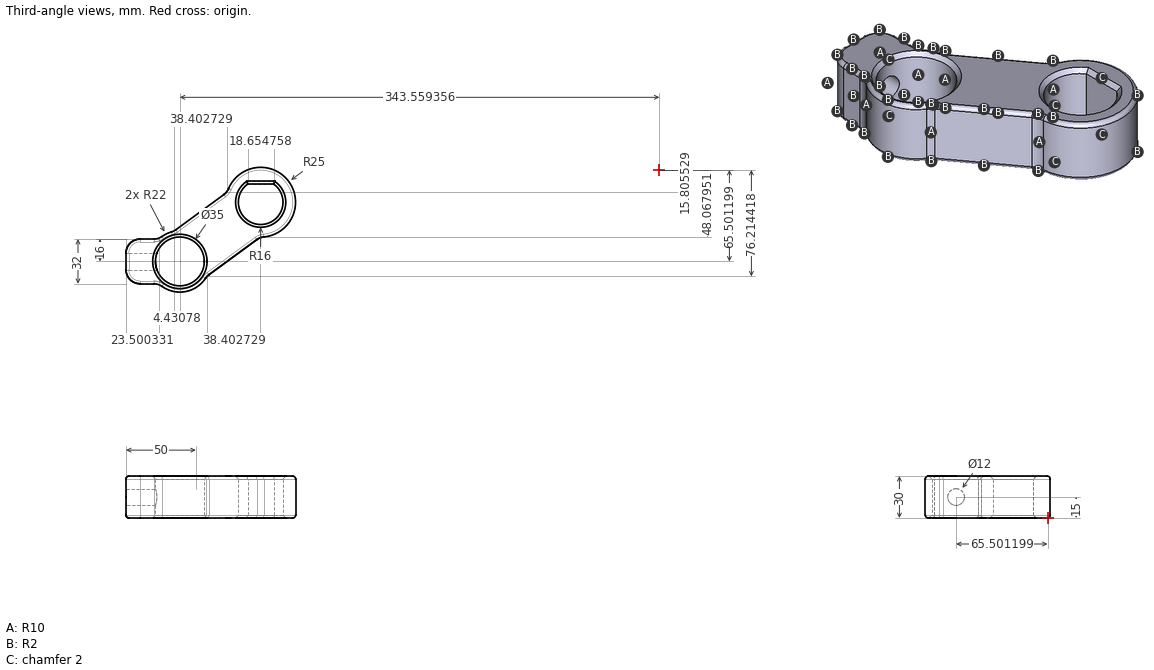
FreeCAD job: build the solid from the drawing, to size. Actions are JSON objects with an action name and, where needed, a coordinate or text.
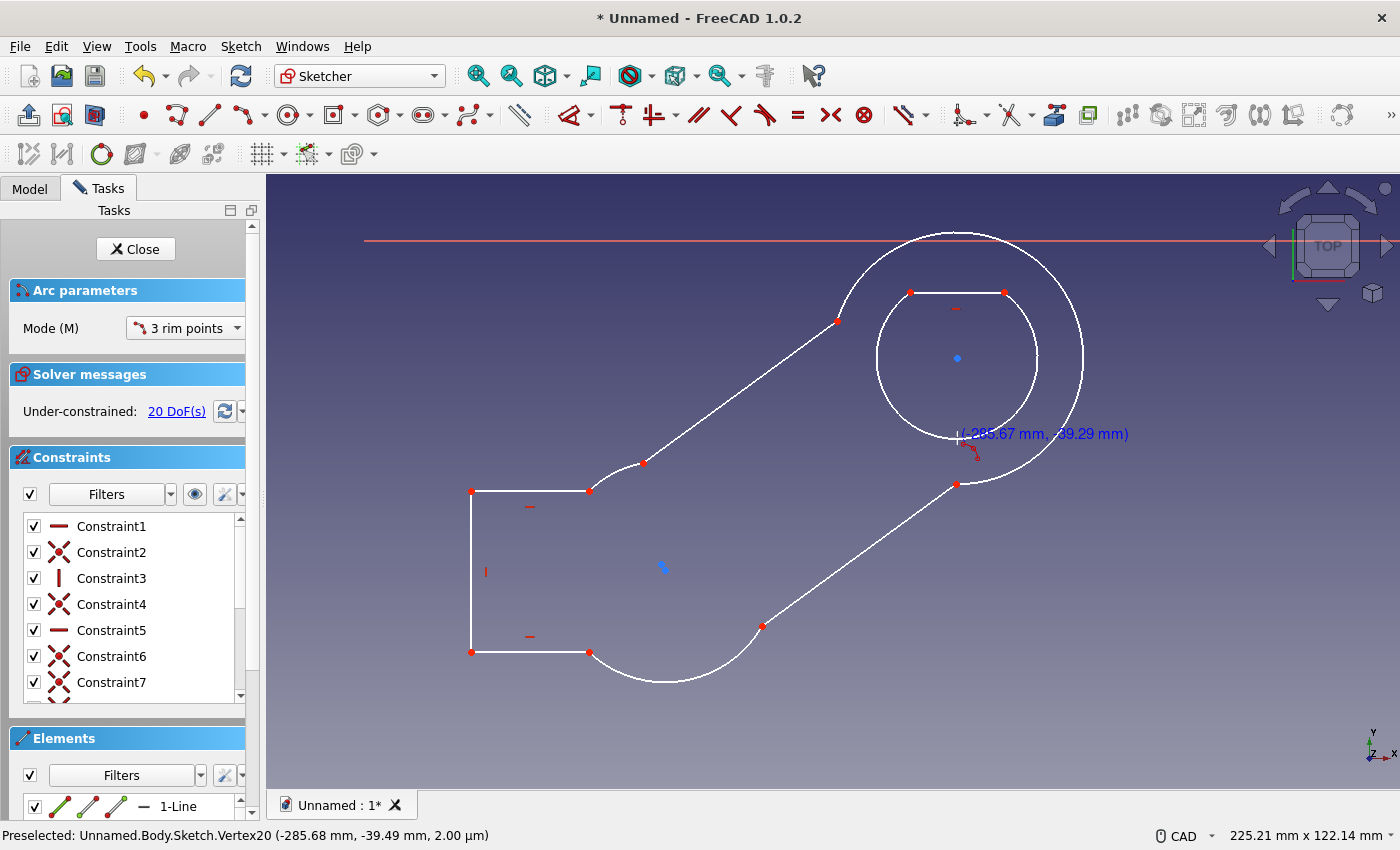
{"action": "left_click", "coordinate": [288, 116]}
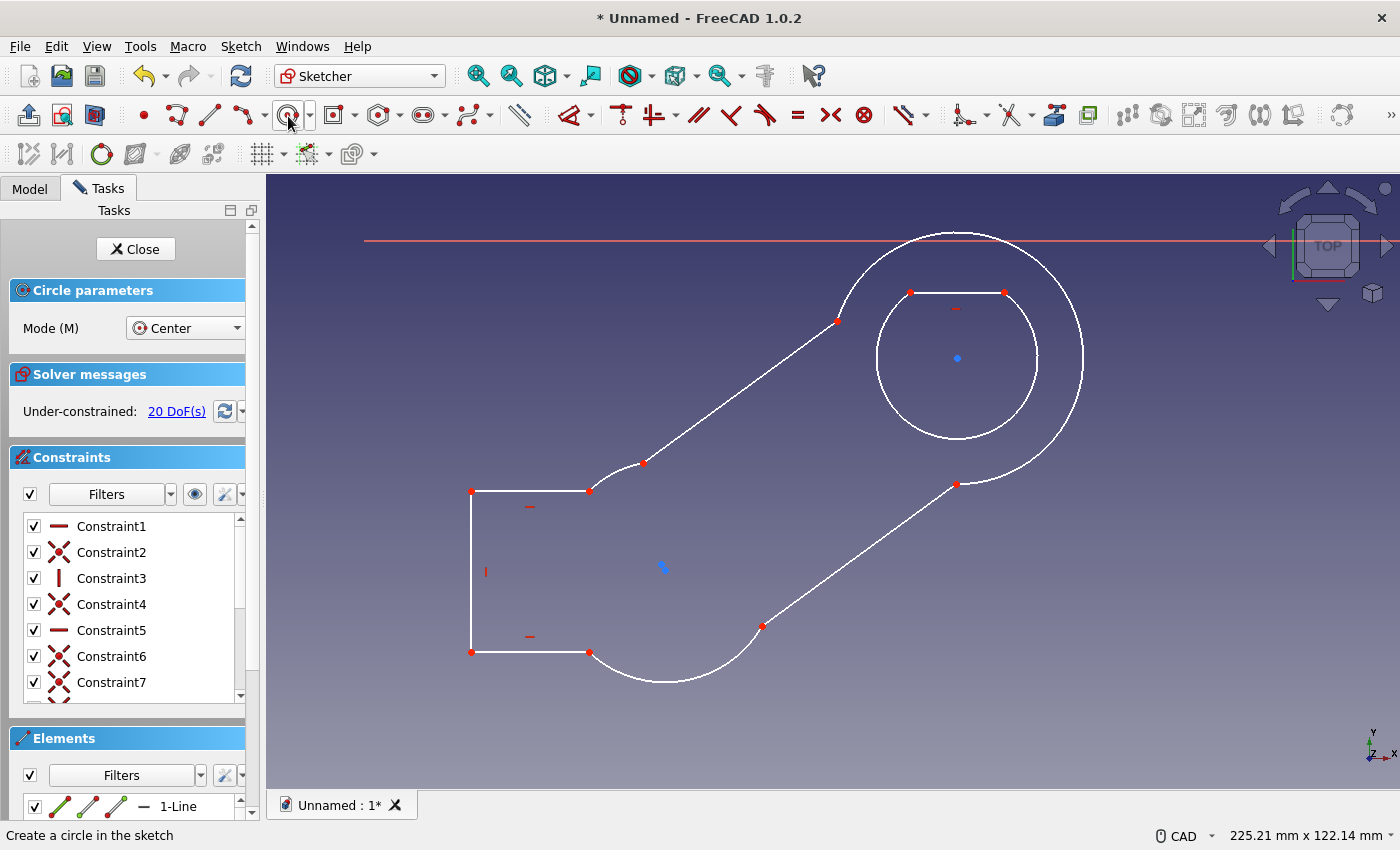
{"action": "left_click", "coordinate": [666, 571]}
{"action": "left_click", "coordinate": [728, 509]}
{"action": "key", "text": "Escape"}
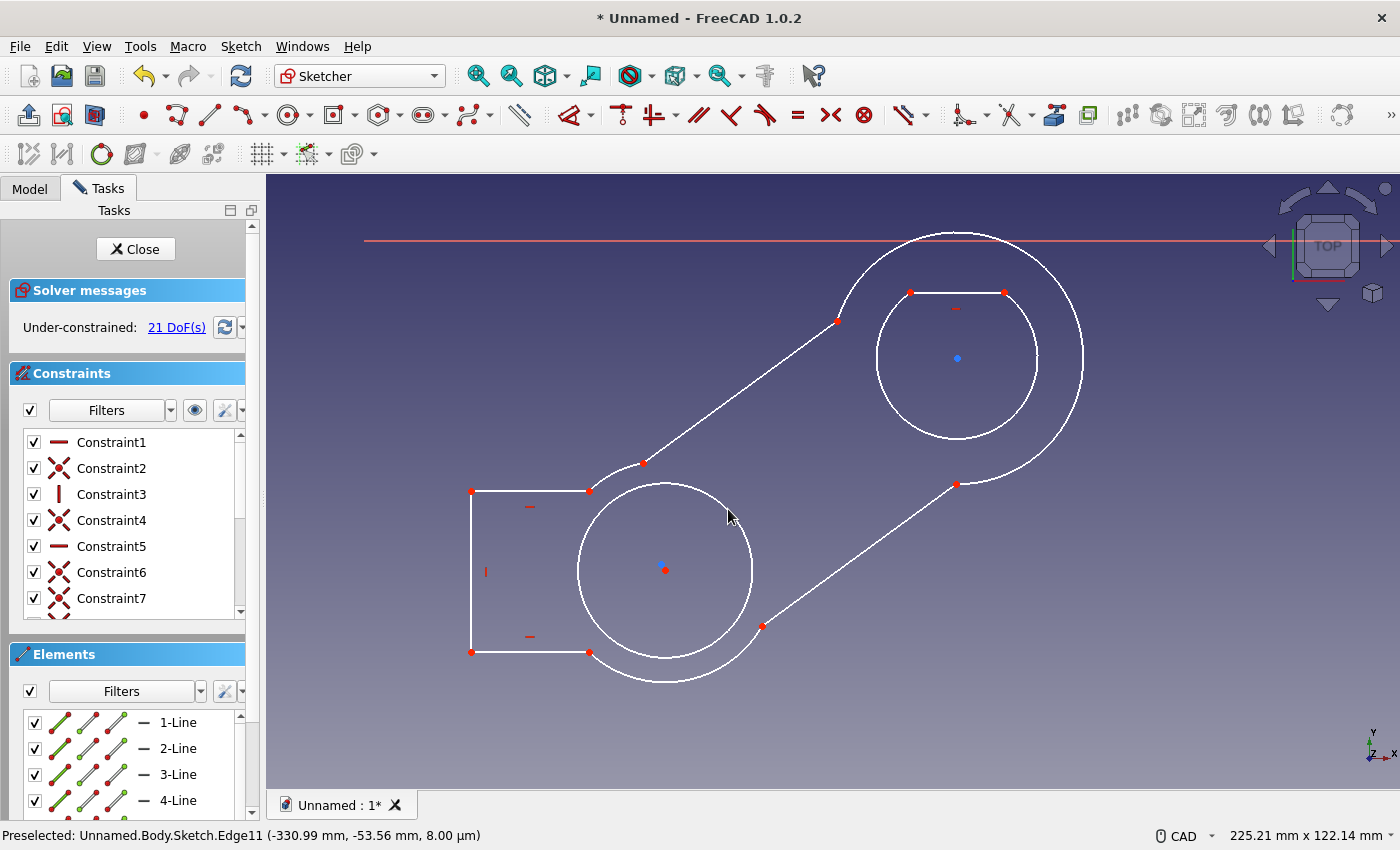
{"action": "left_click", "coordinate": [727, 509]}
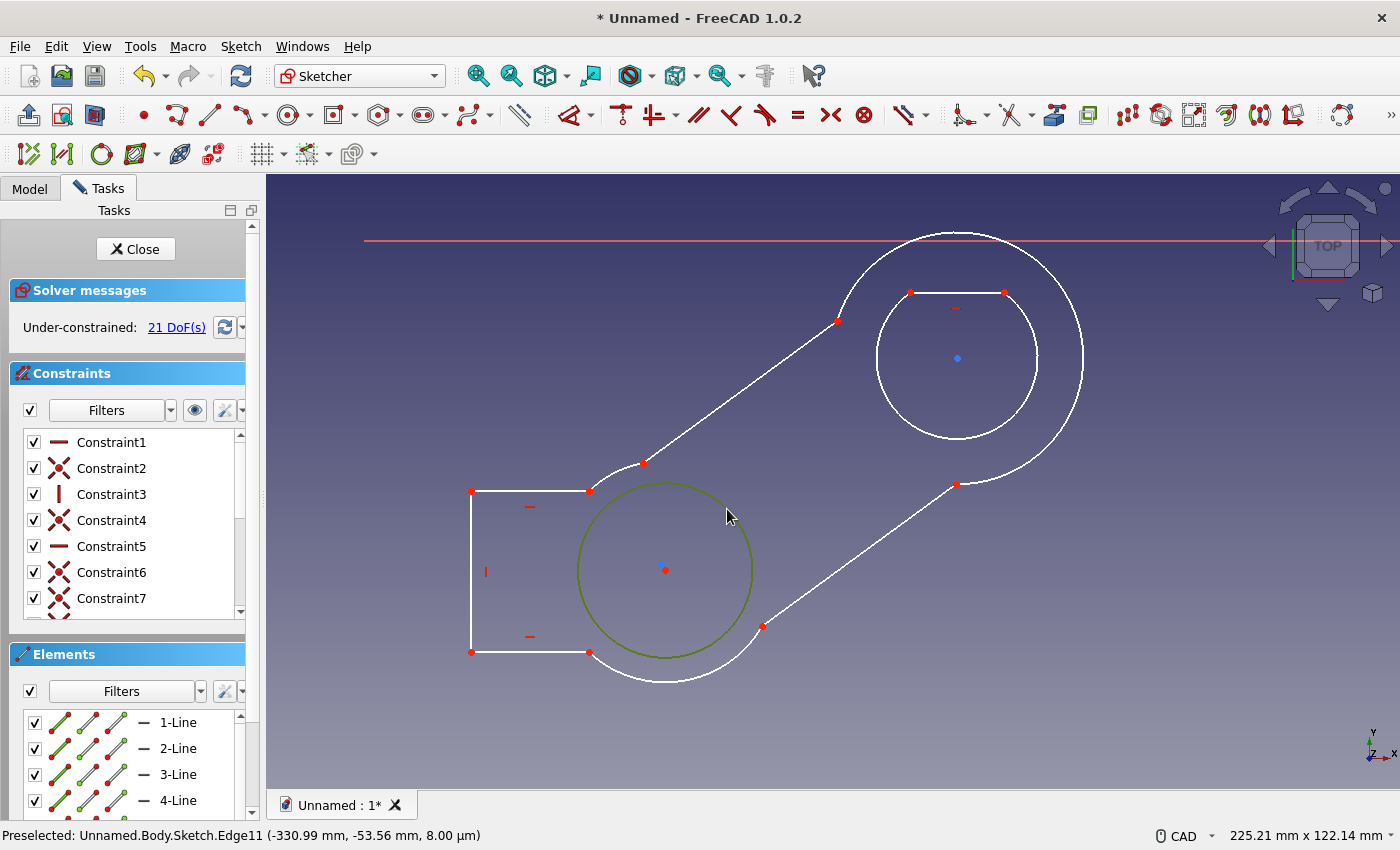
{"action": "left_click", "coordinate": [625, 468]}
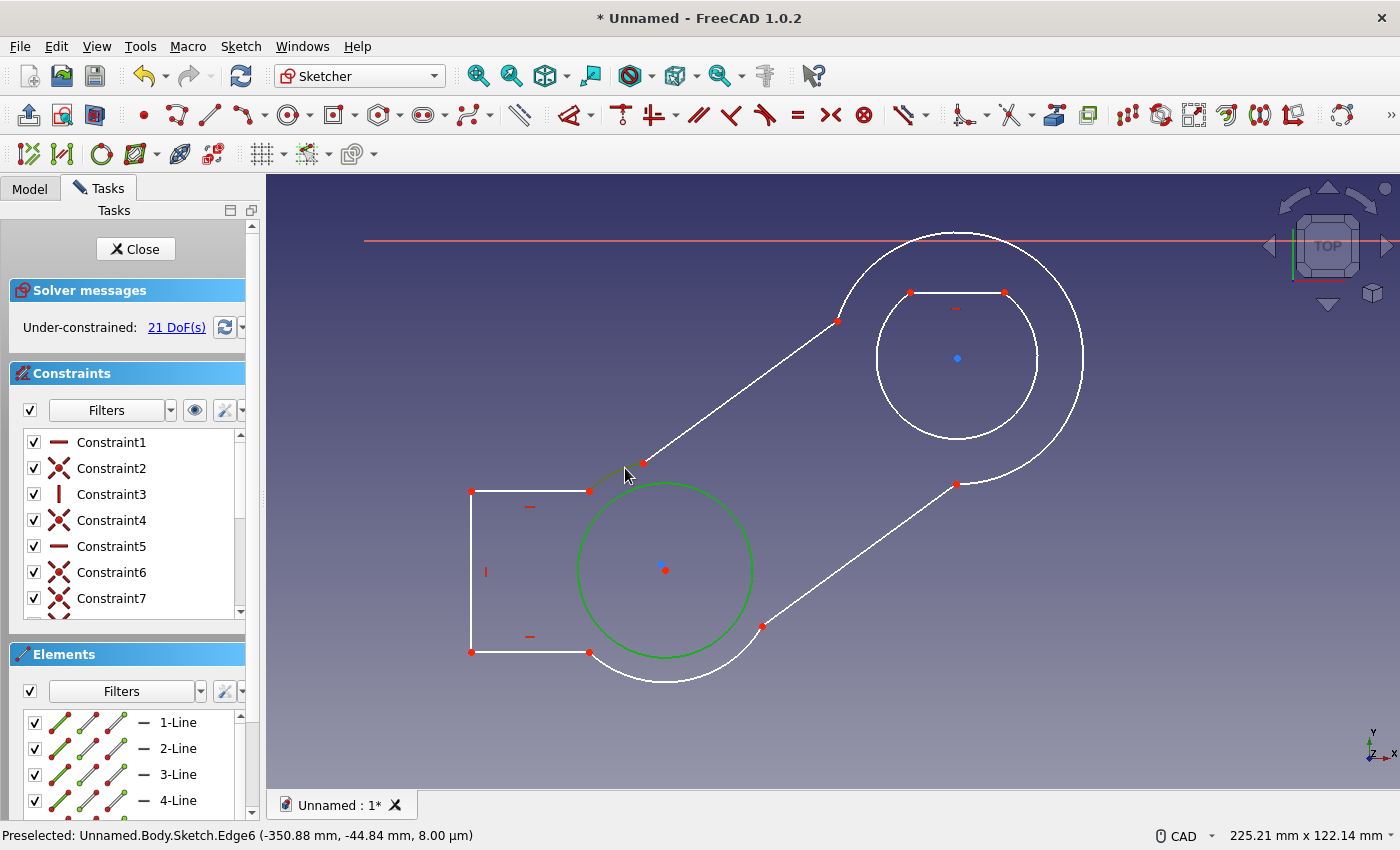
{"action": "left_click", "coordinate": [621, 116]}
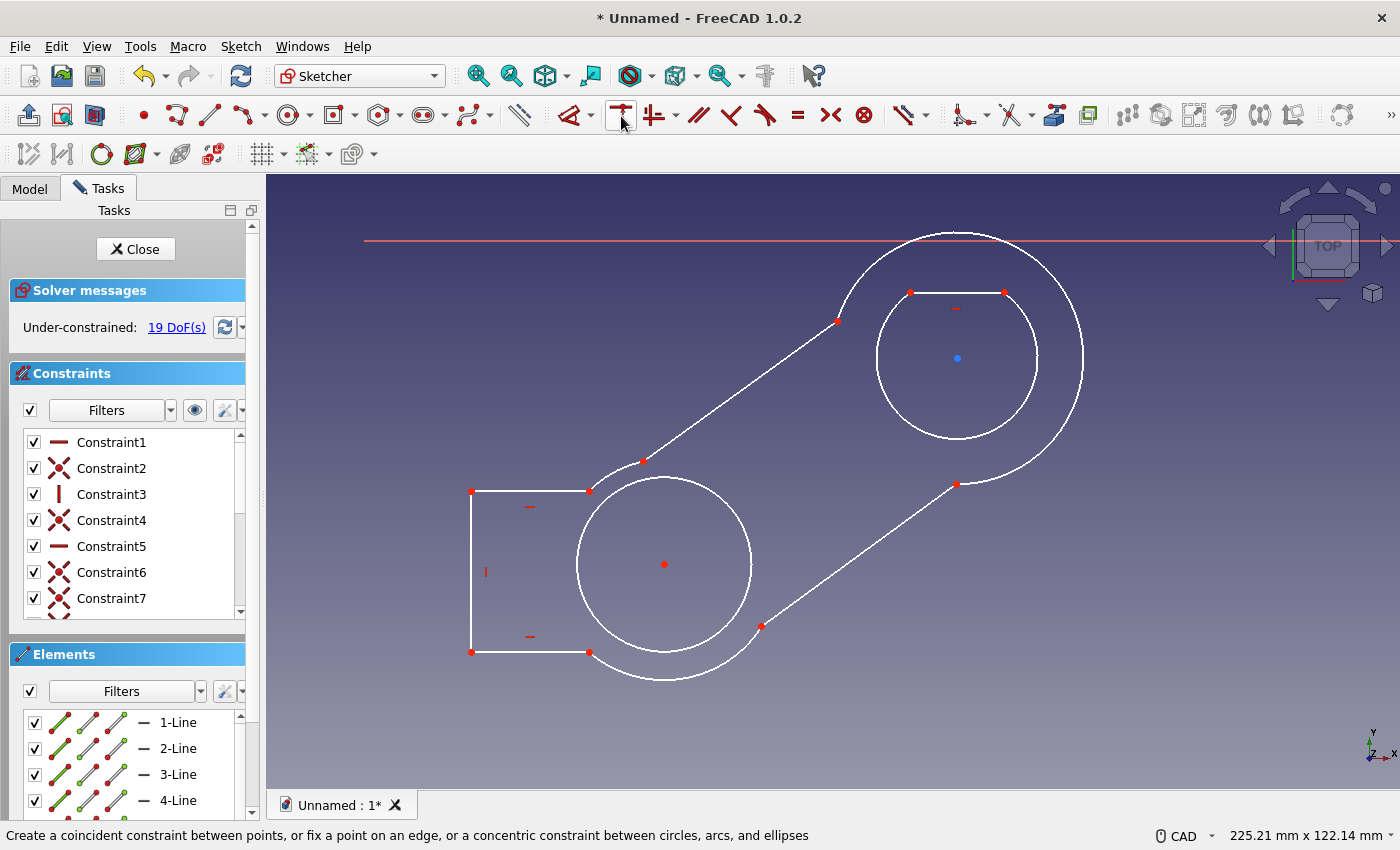
{"action": "left_click", "coordinate": [1079, 390]}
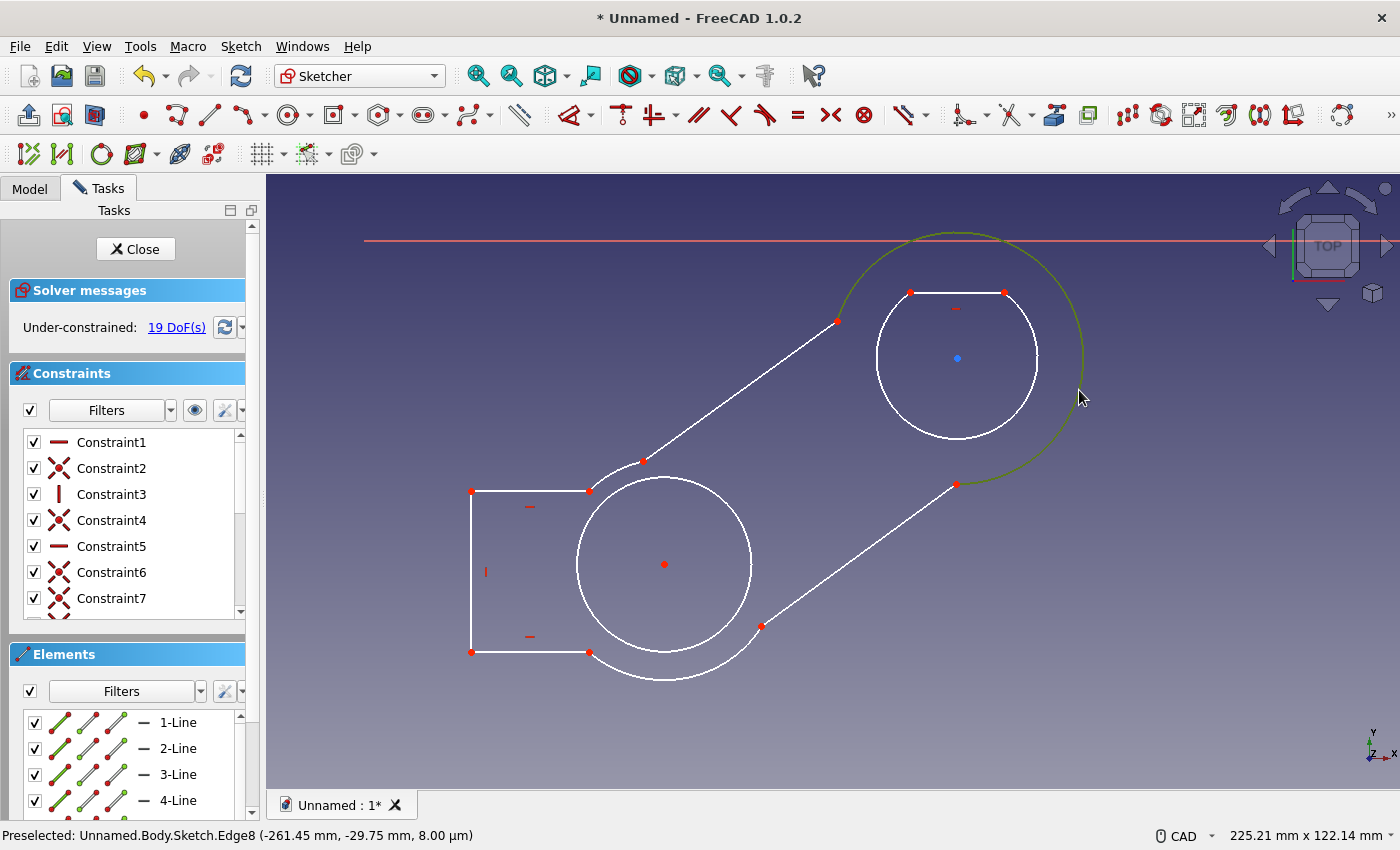
{"action": "left_click", "coordinate": [889, 401]}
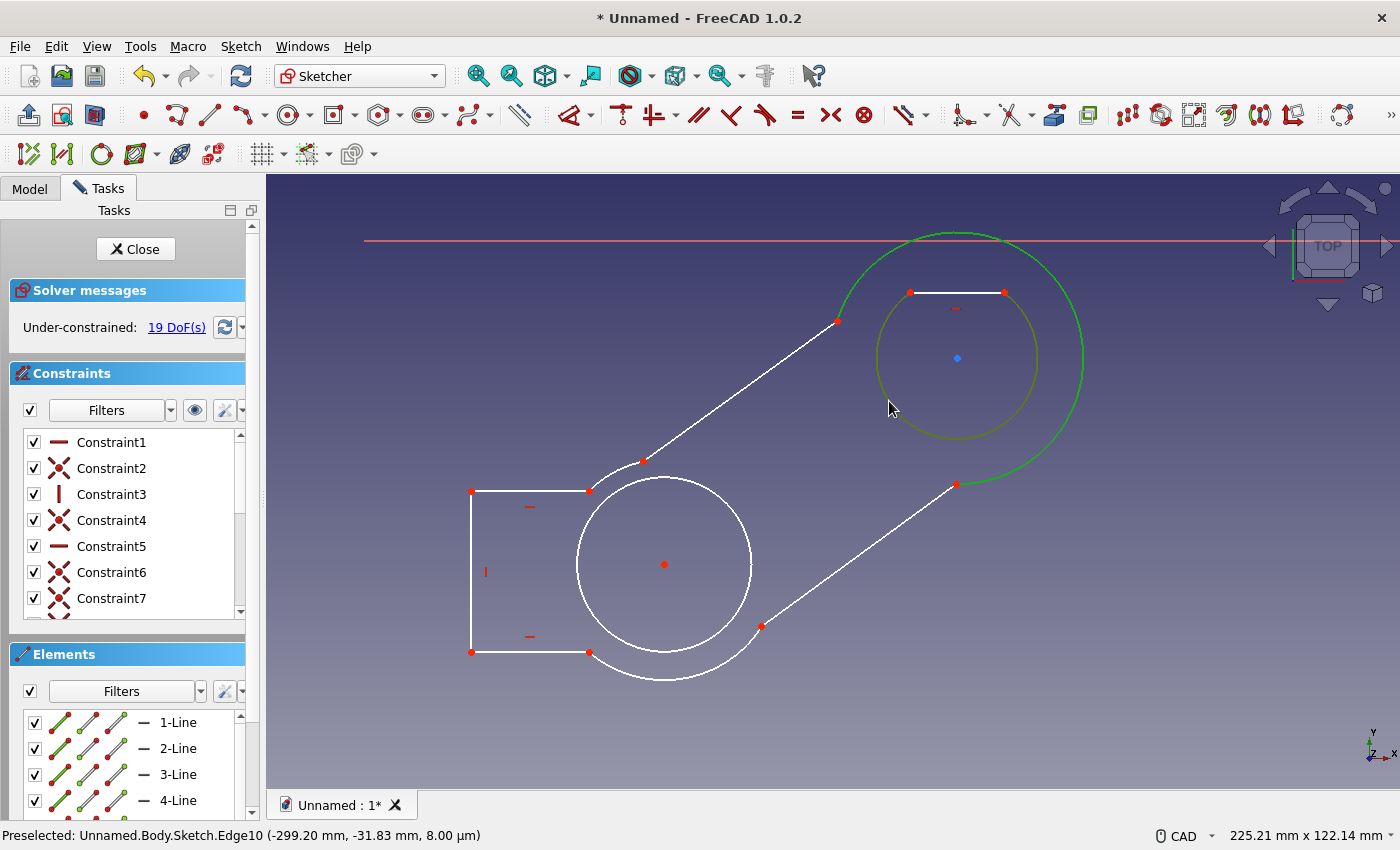
{"action": "left_click", "coordinate": [621, 116]}